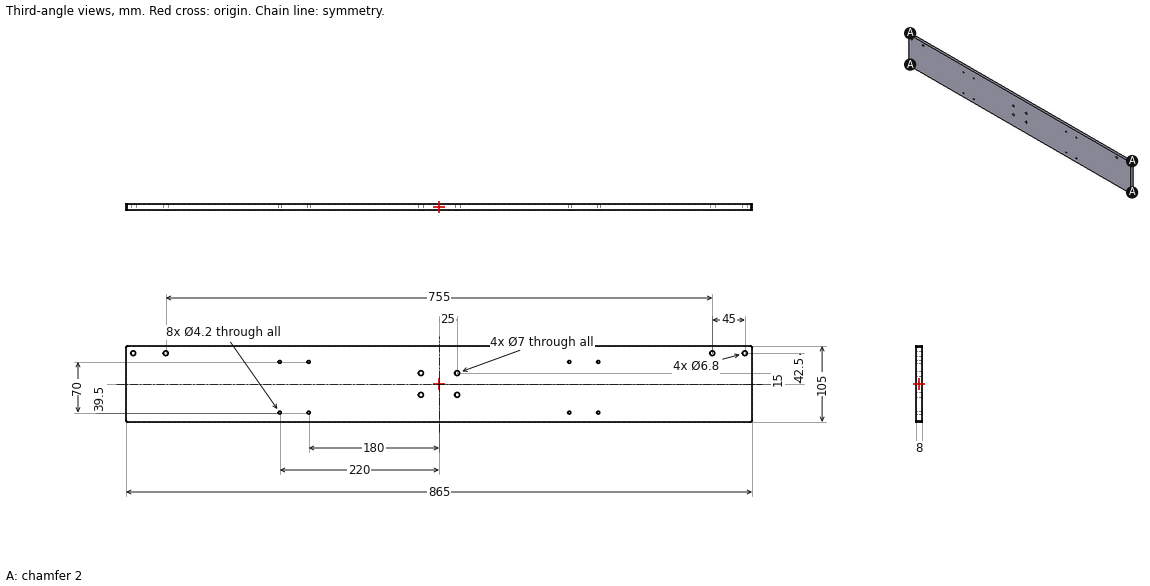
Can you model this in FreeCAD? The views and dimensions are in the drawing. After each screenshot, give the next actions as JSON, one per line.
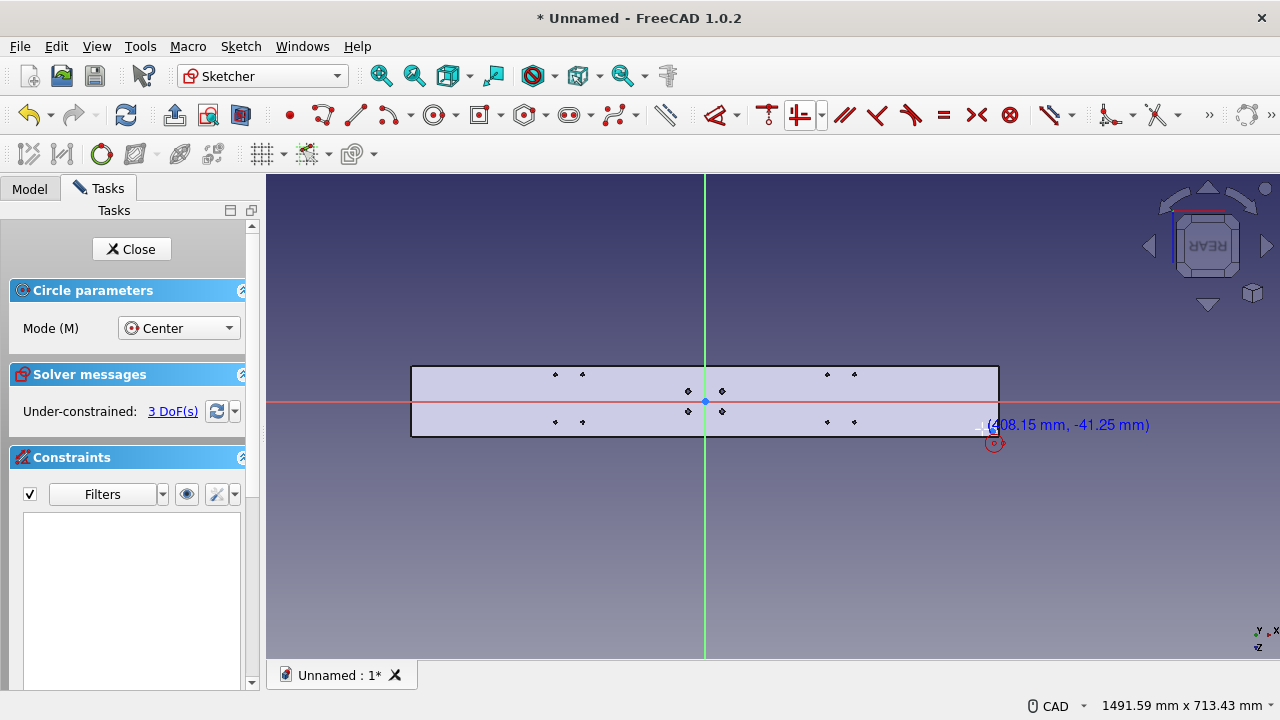
{"action": "left_click", "coordinate": [962, 430]}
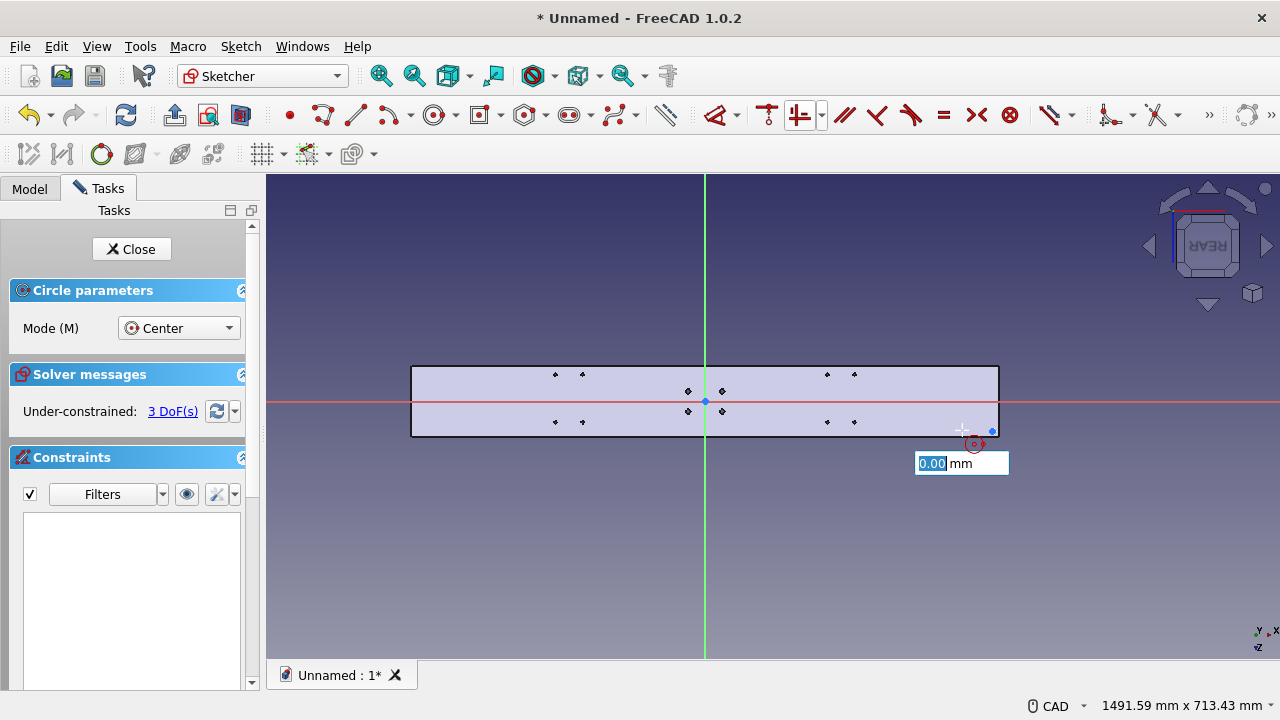
{"action": "scroll", "coordinate": [963, 429], "scroll_direction": "up", "scroll_amount": 10}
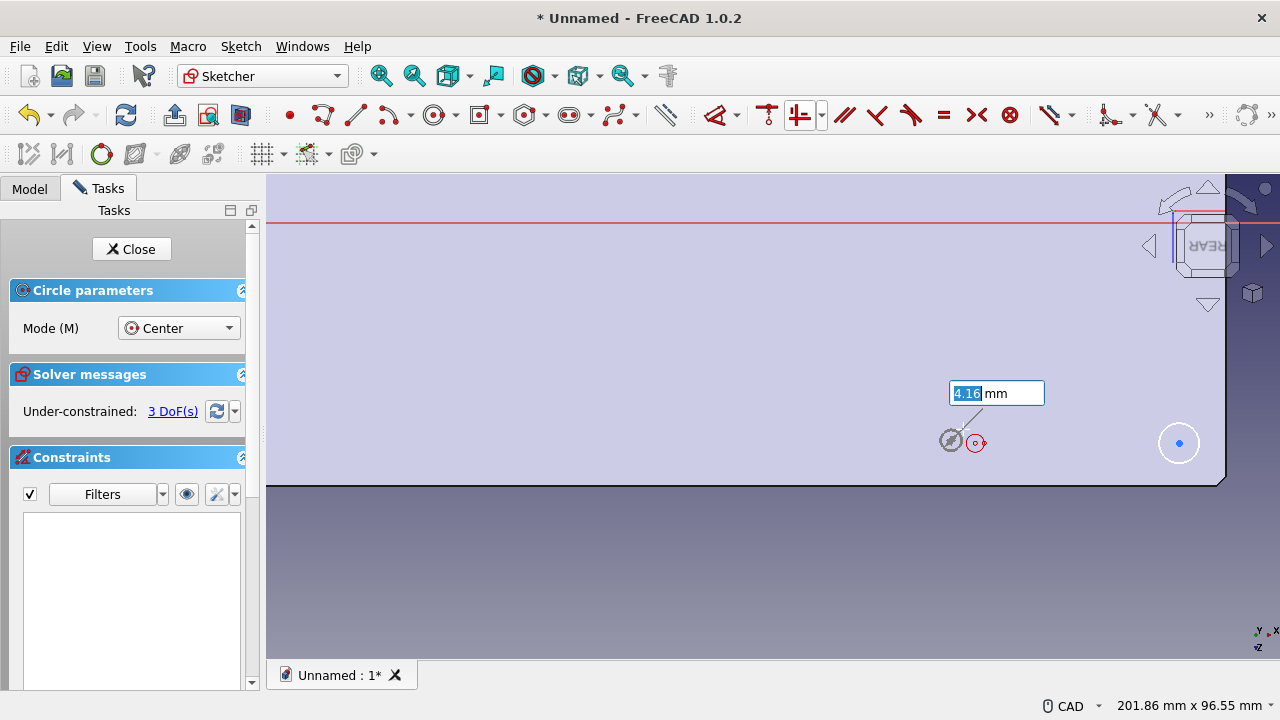
{"action": "left_click", "coordinate": [962, 424]}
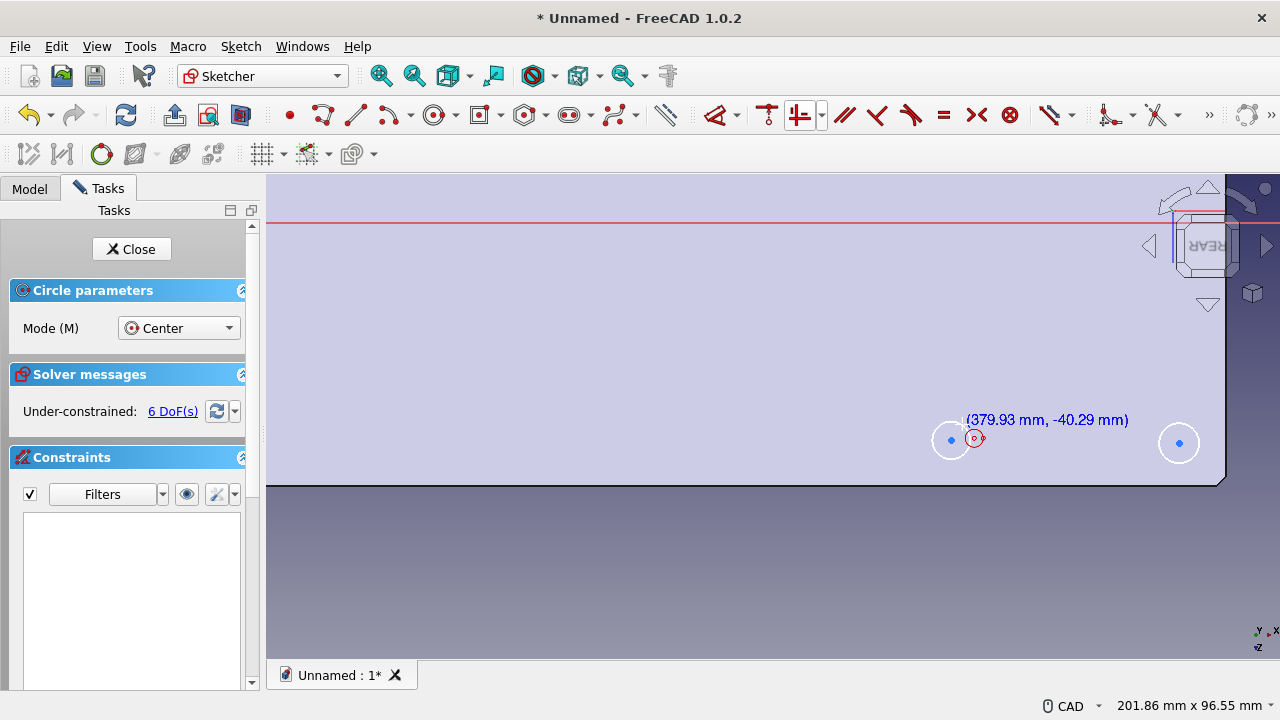
{"action": "scroll", "coordinate": [963, 429], "scroll_direction": "down", "scroll_amount": 10}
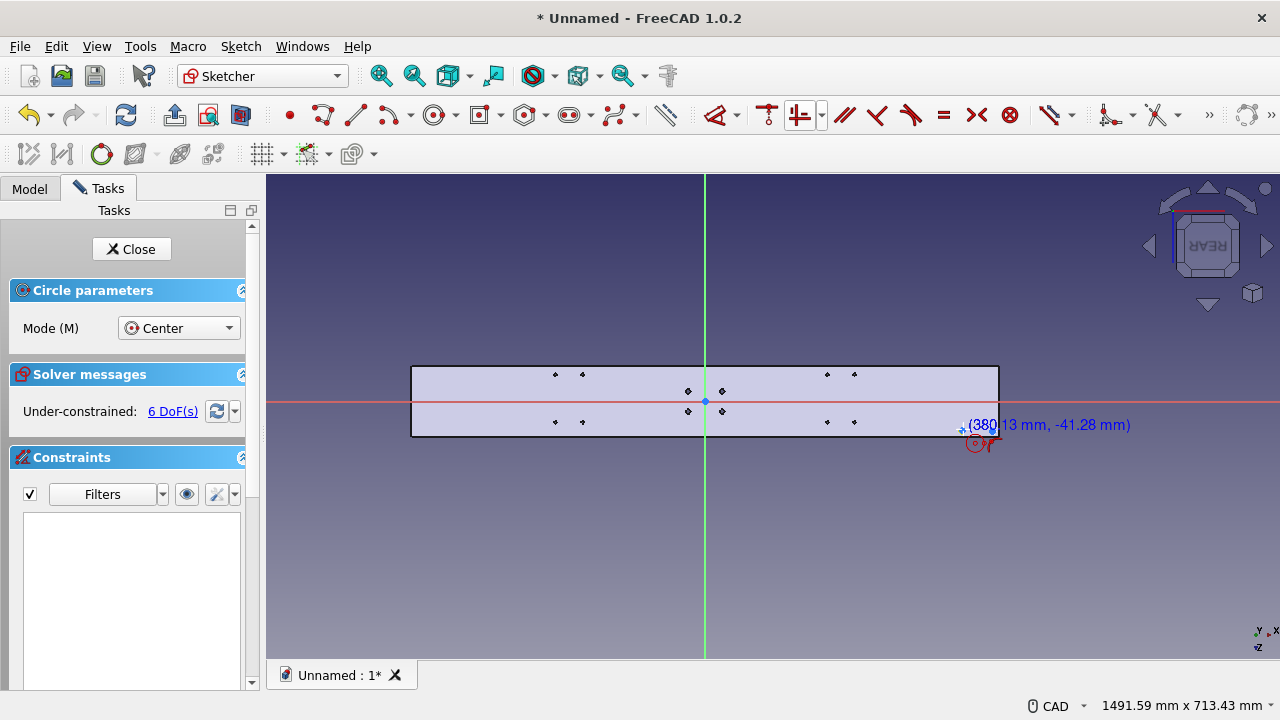
{"action": "scroll", "coordinate": [449, 430], "scroll_direction": "up", "scroll_amount": 12}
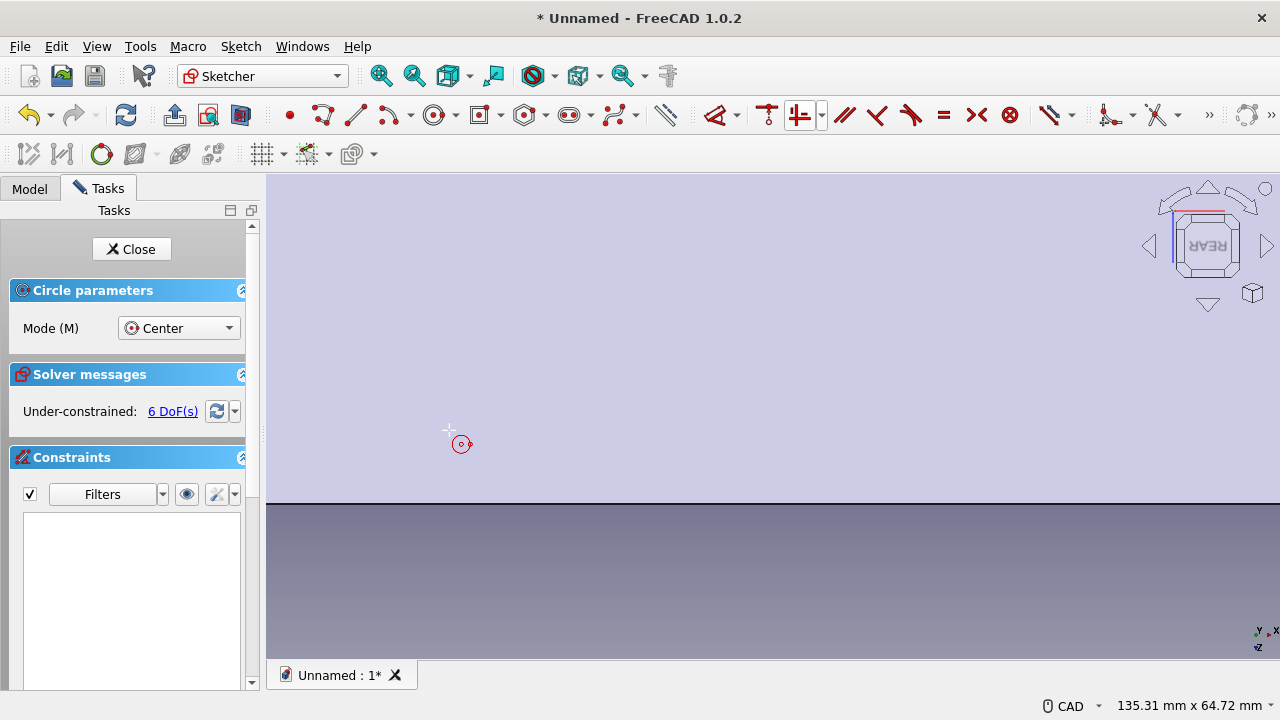
{"action": "scroll", "coordinate": [448, 430], "scroll_direction": "down", "scroll_amount": 12}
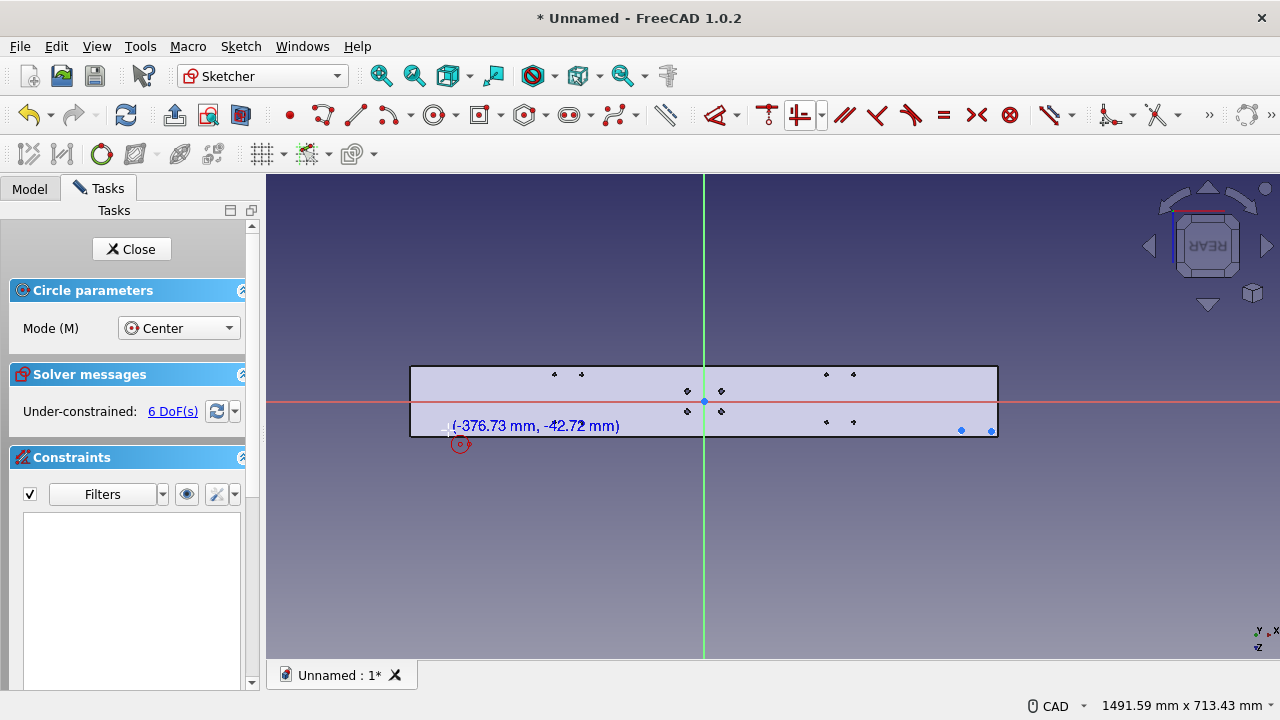
{"action": "left_click", "coordinate": [448, 430]}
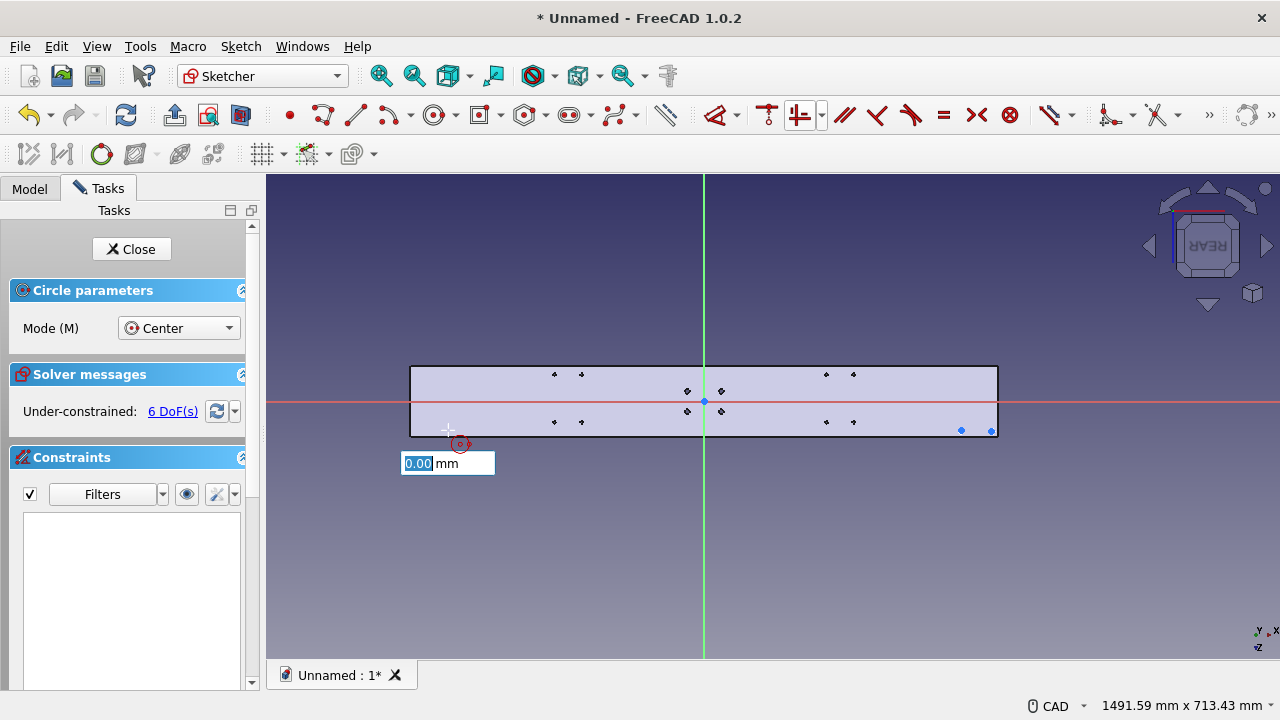
{"action": "scroll", "coordinate": [449, 429], "scroll_direction": "up", "scroll_amount": 10}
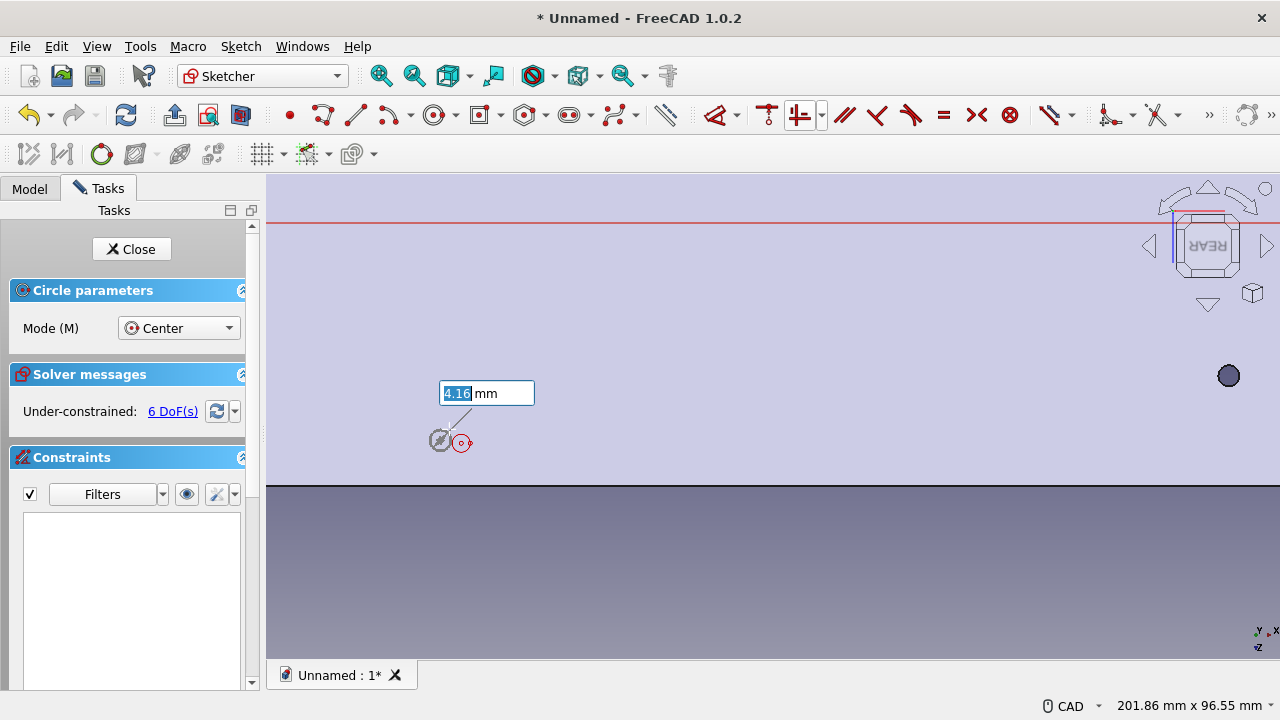
{"action": "left_click", "coordinate": [450, 424]}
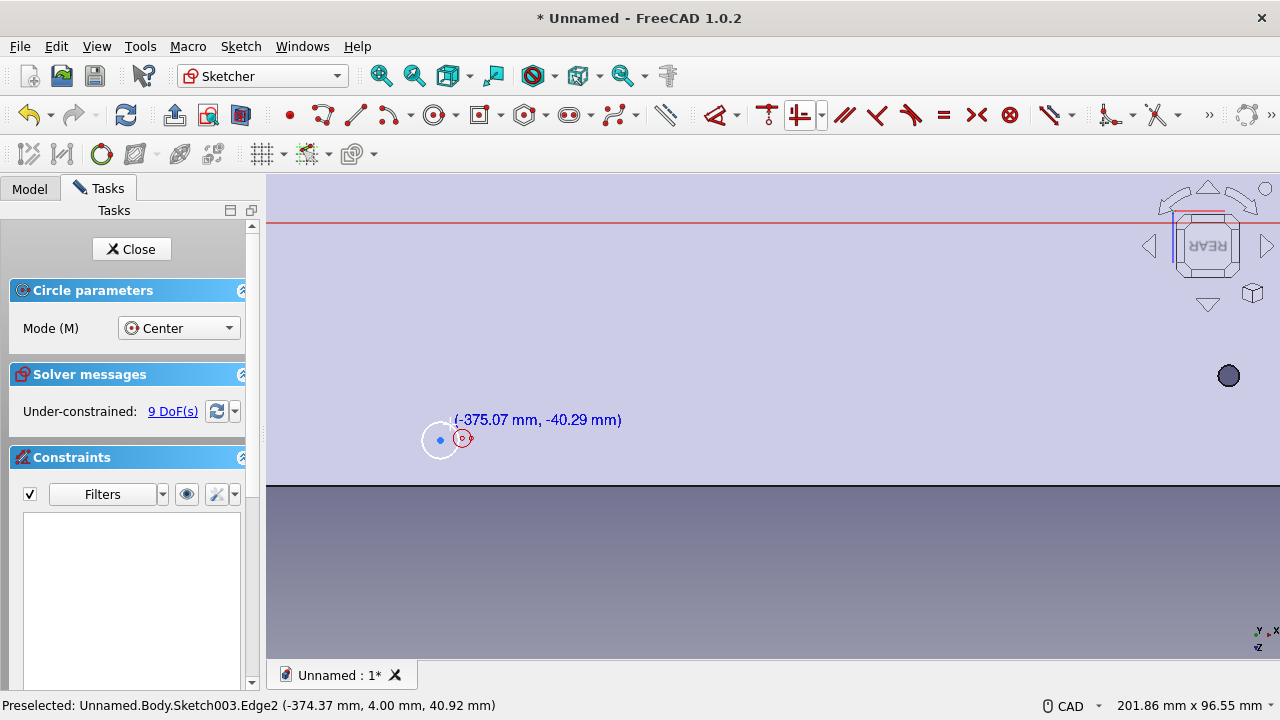
{"action": "scroll", "coordinate": [449, 429], "scroll_direction": "down", "scroll_amount": 10}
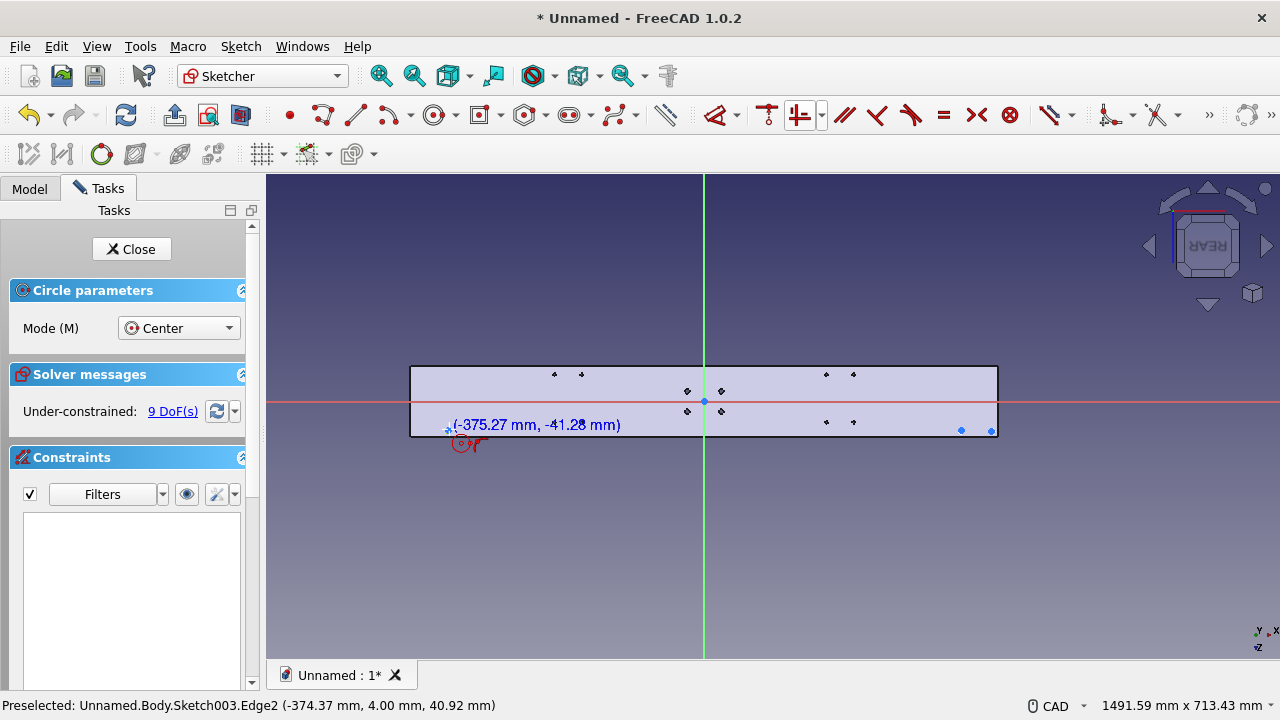
{"action": "scroll", "coordinate": [417, 430], "scroll_direction": "up", "scroll_amount": 12}